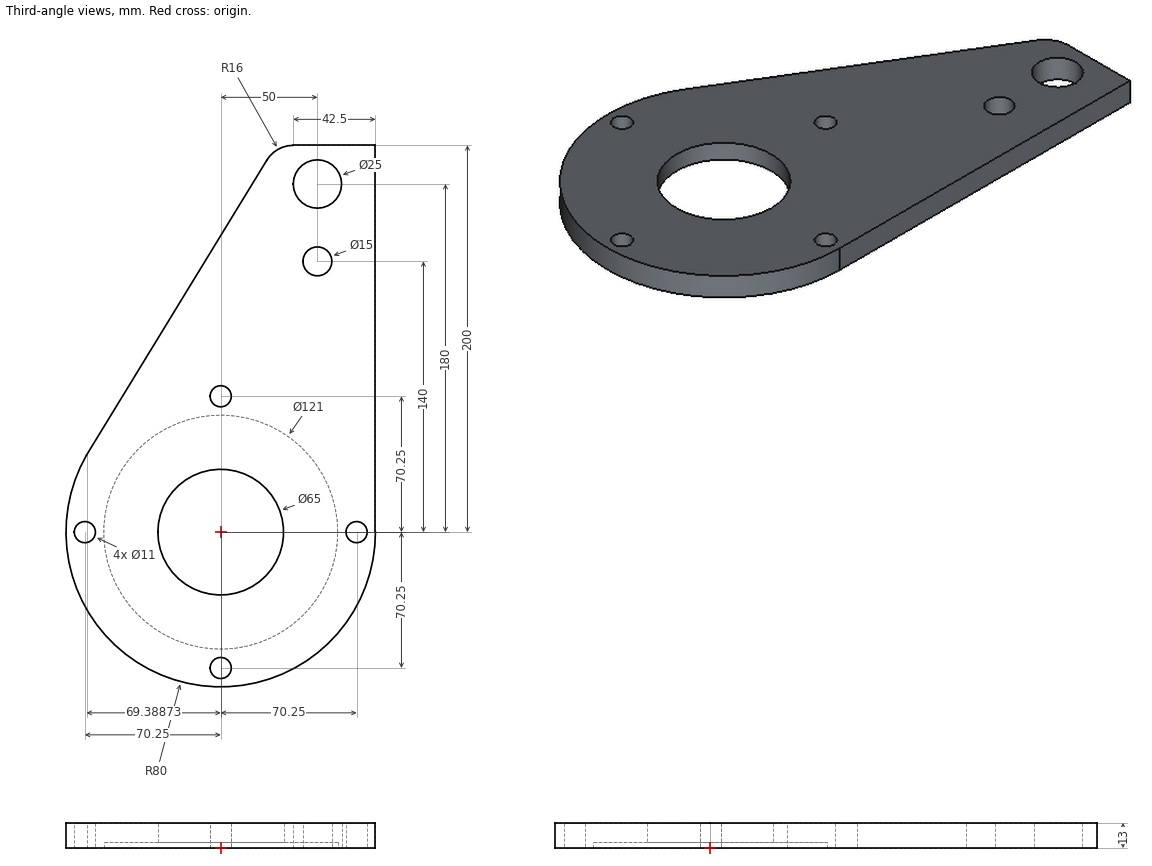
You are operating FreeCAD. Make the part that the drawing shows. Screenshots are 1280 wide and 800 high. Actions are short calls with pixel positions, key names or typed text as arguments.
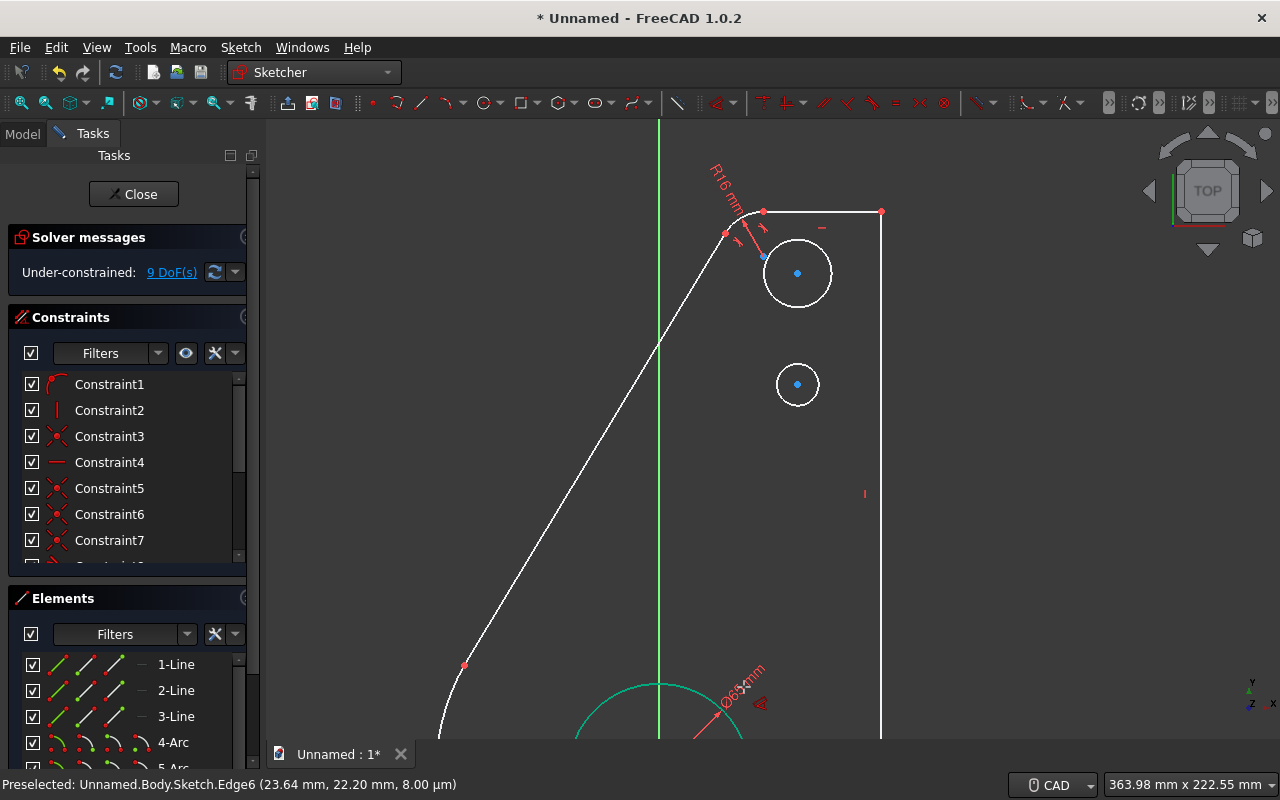
click(812, 370)
click(834, 347)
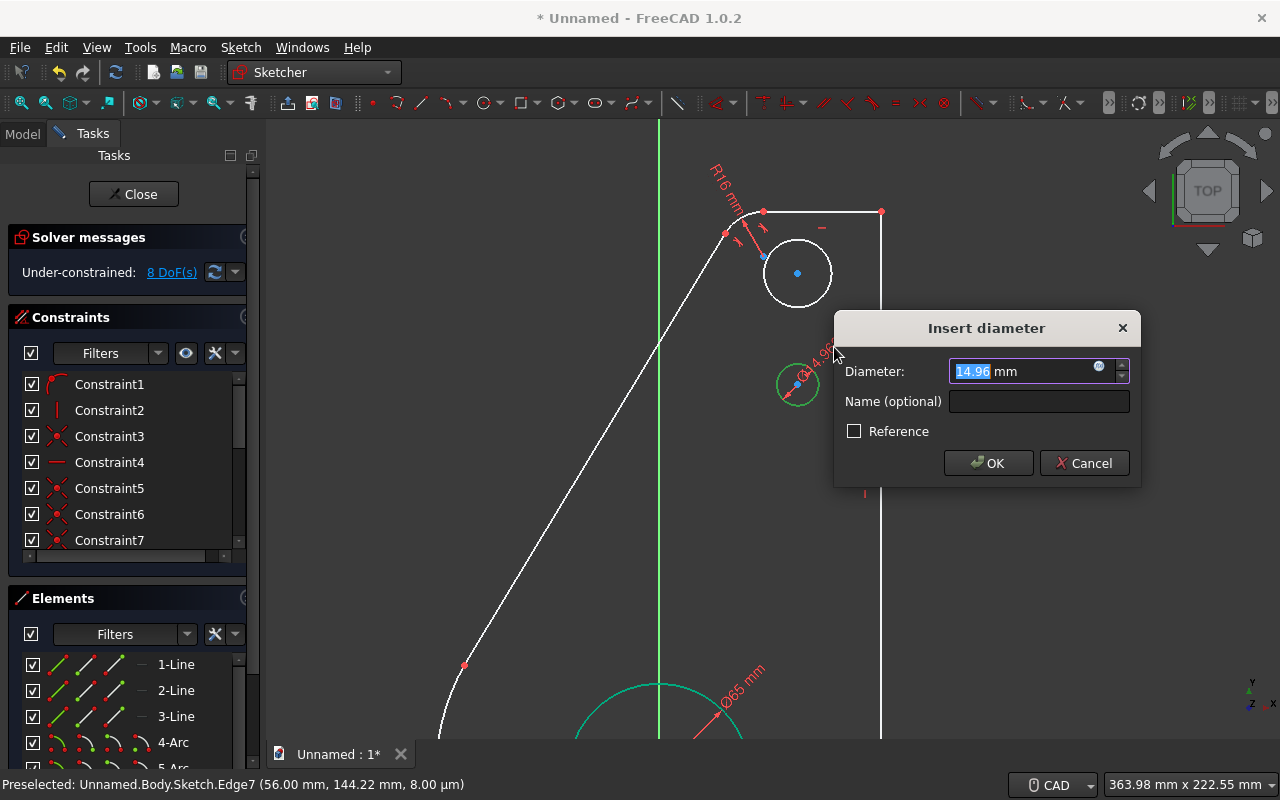
text(15)
key(Return)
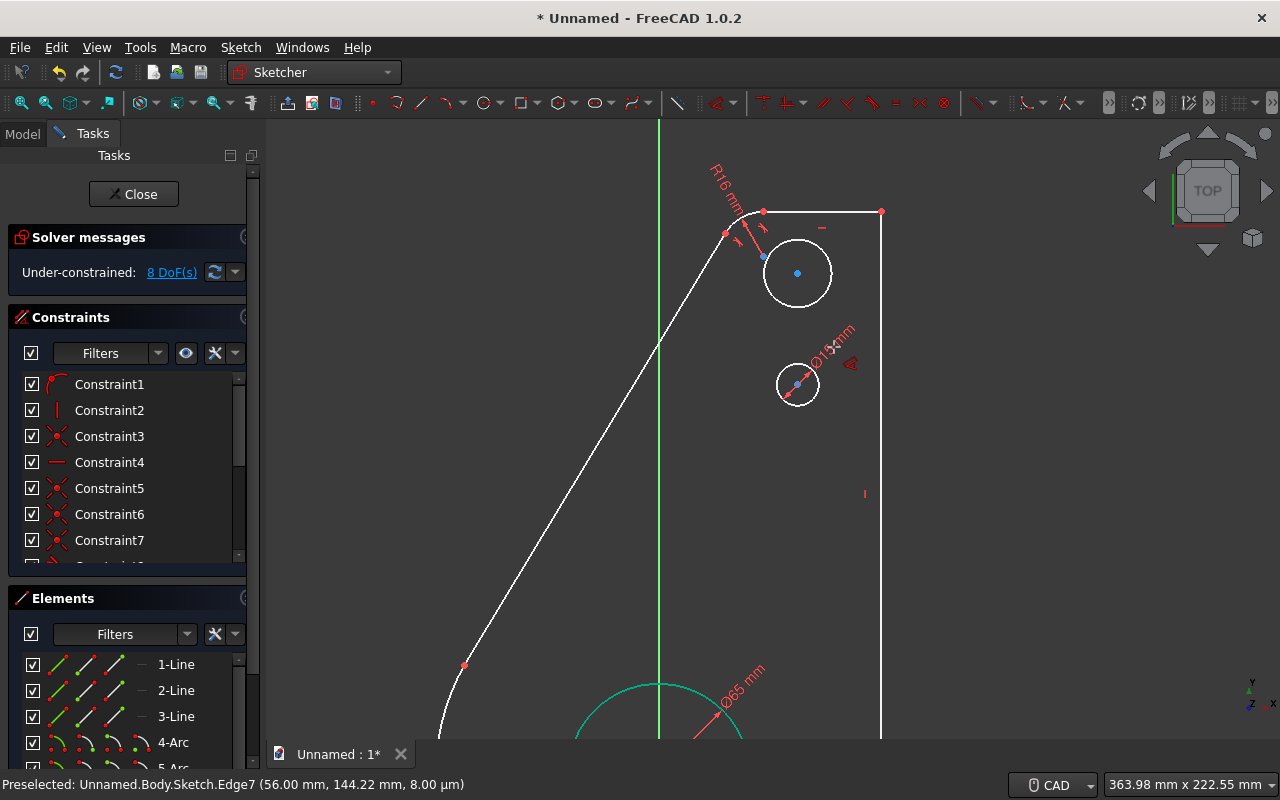
click(822, 249)
click(845, 226)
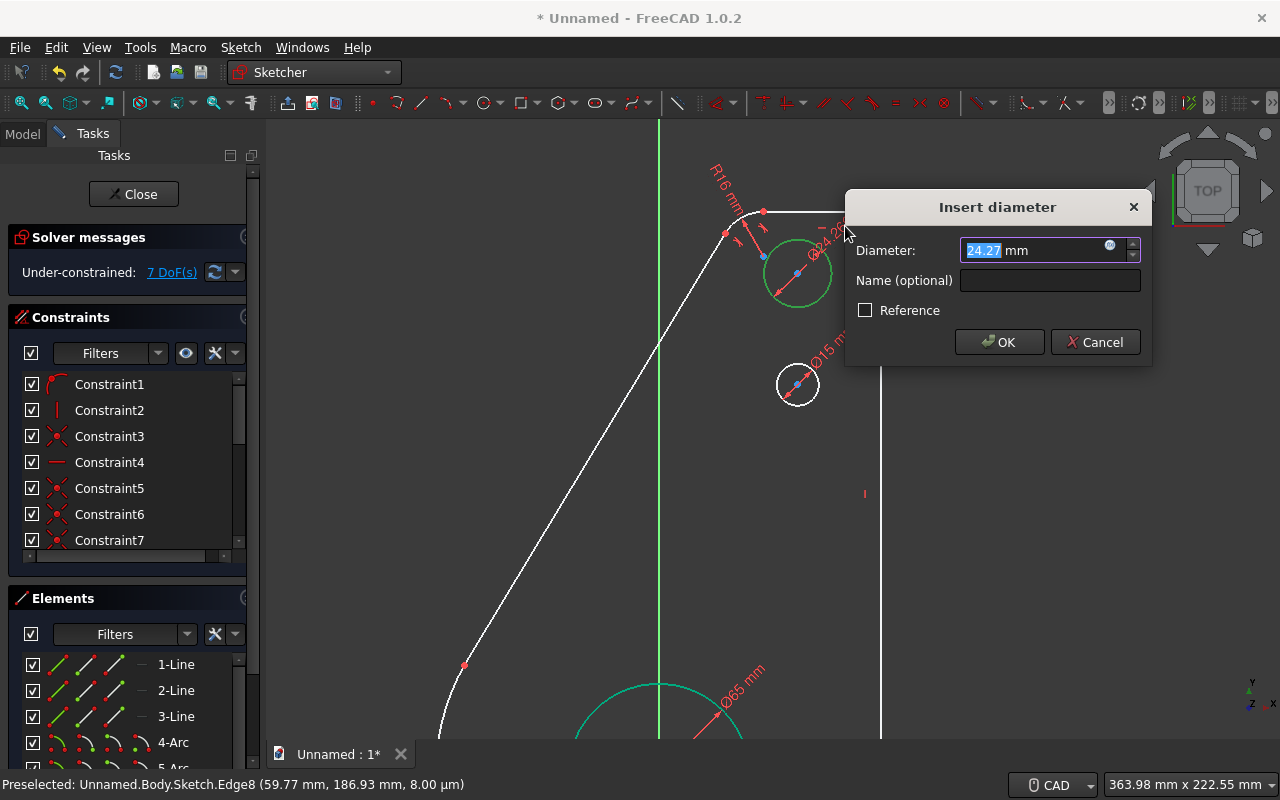
text(25)
key(Return)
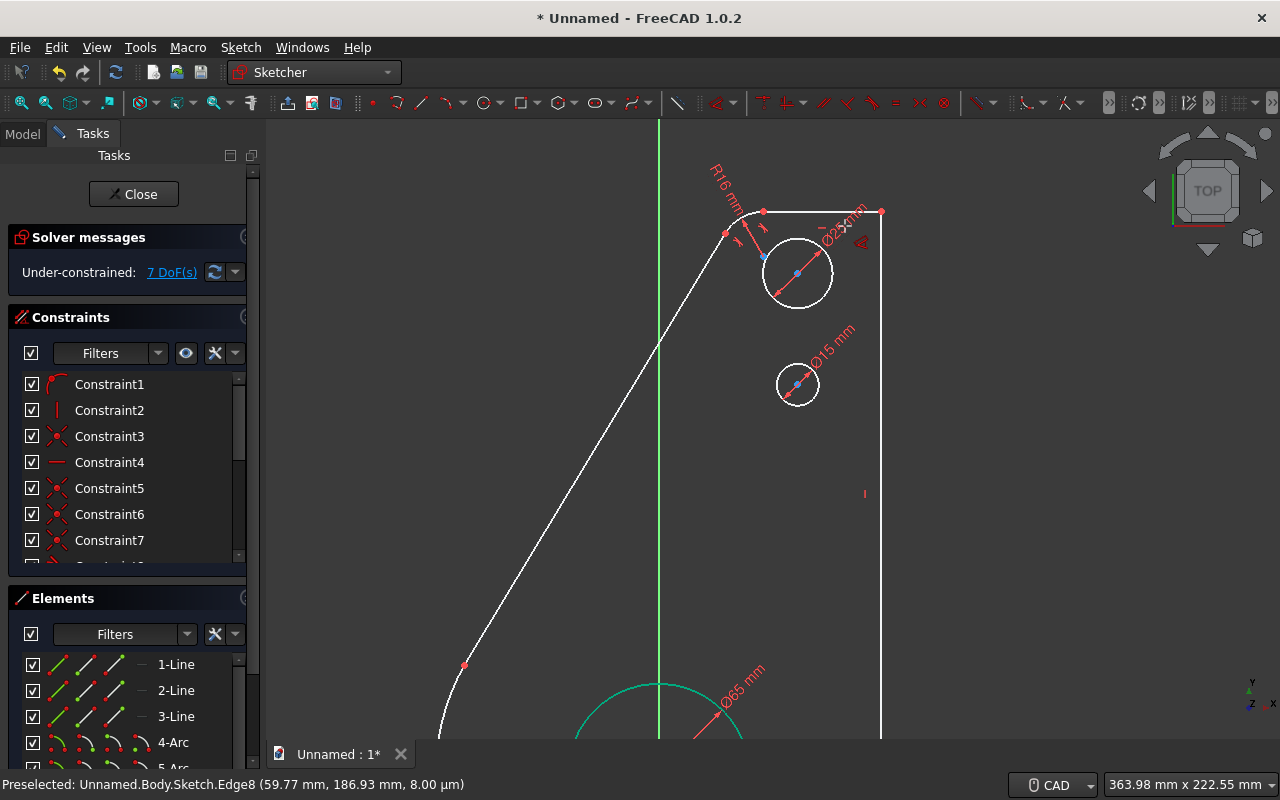
click(798, 385)
click(728, 351)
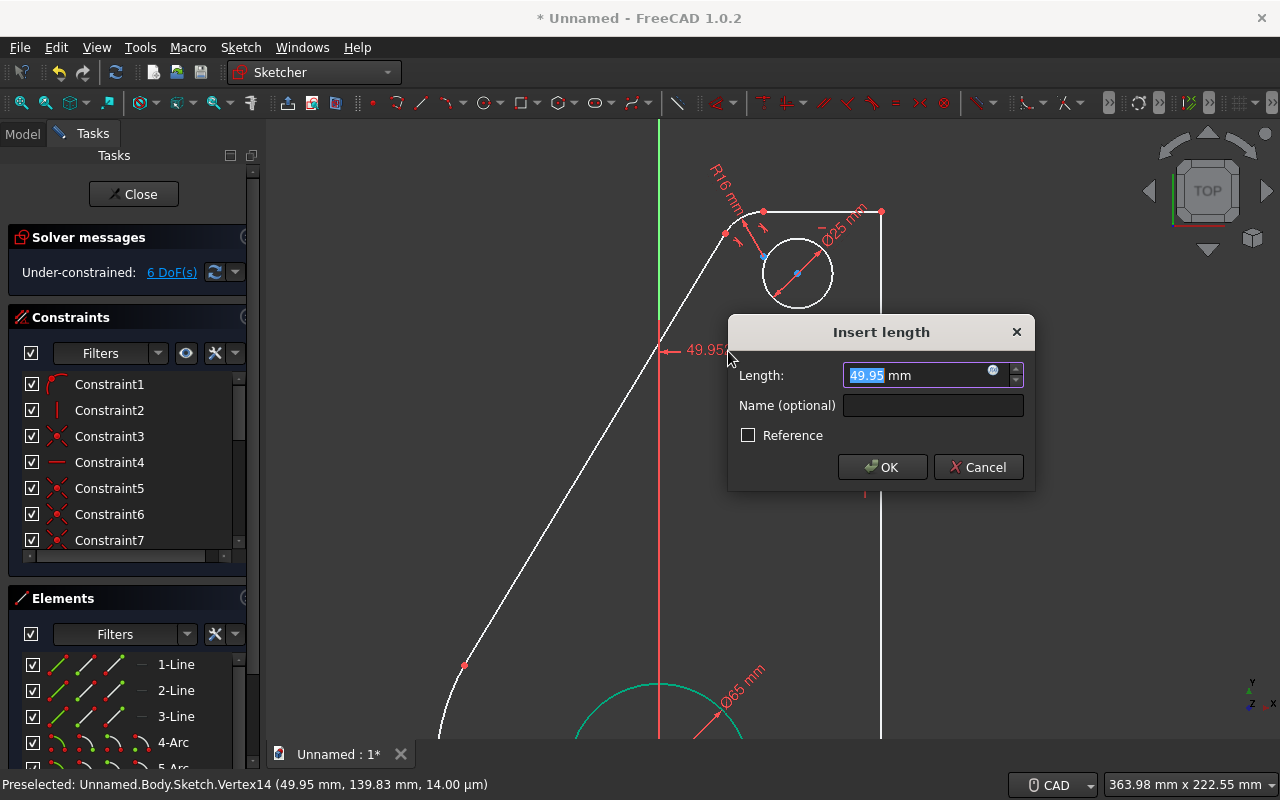
text(50)
key(Return)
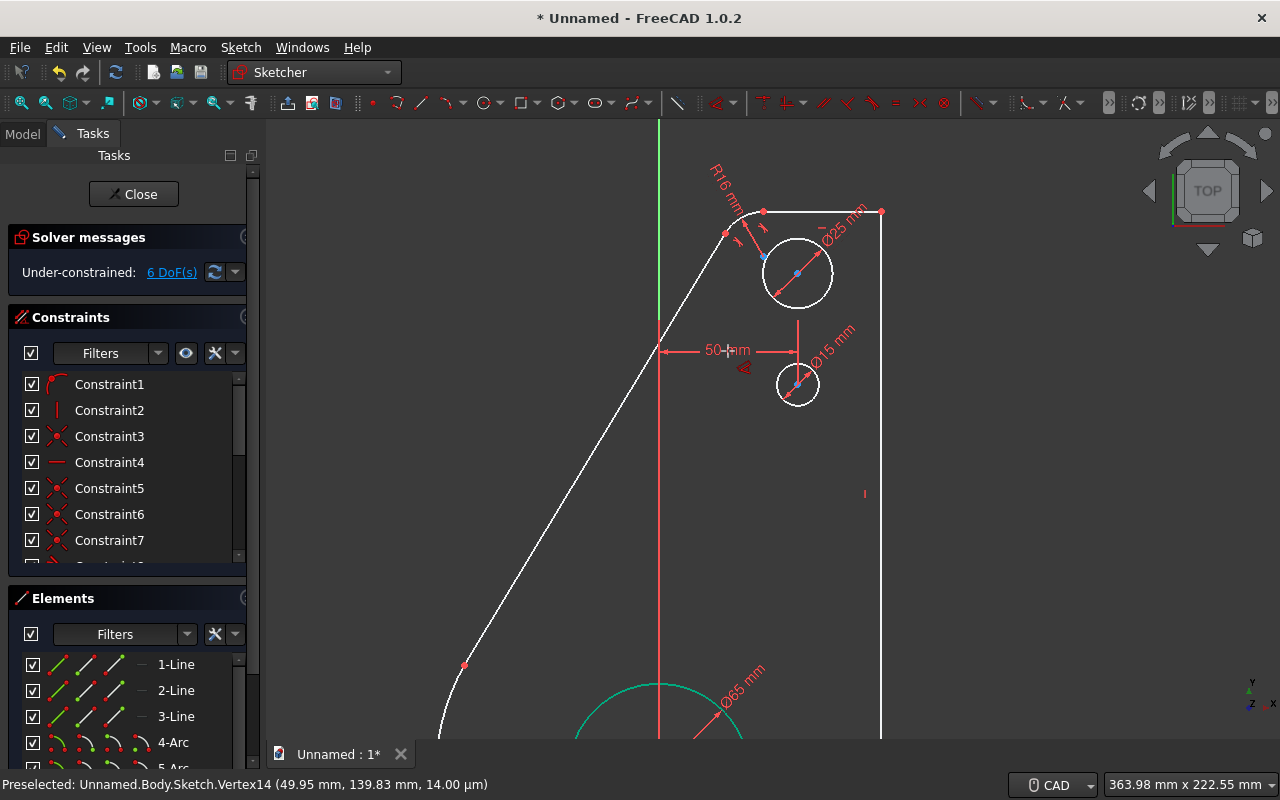
click(798, 273)
click(696, 239)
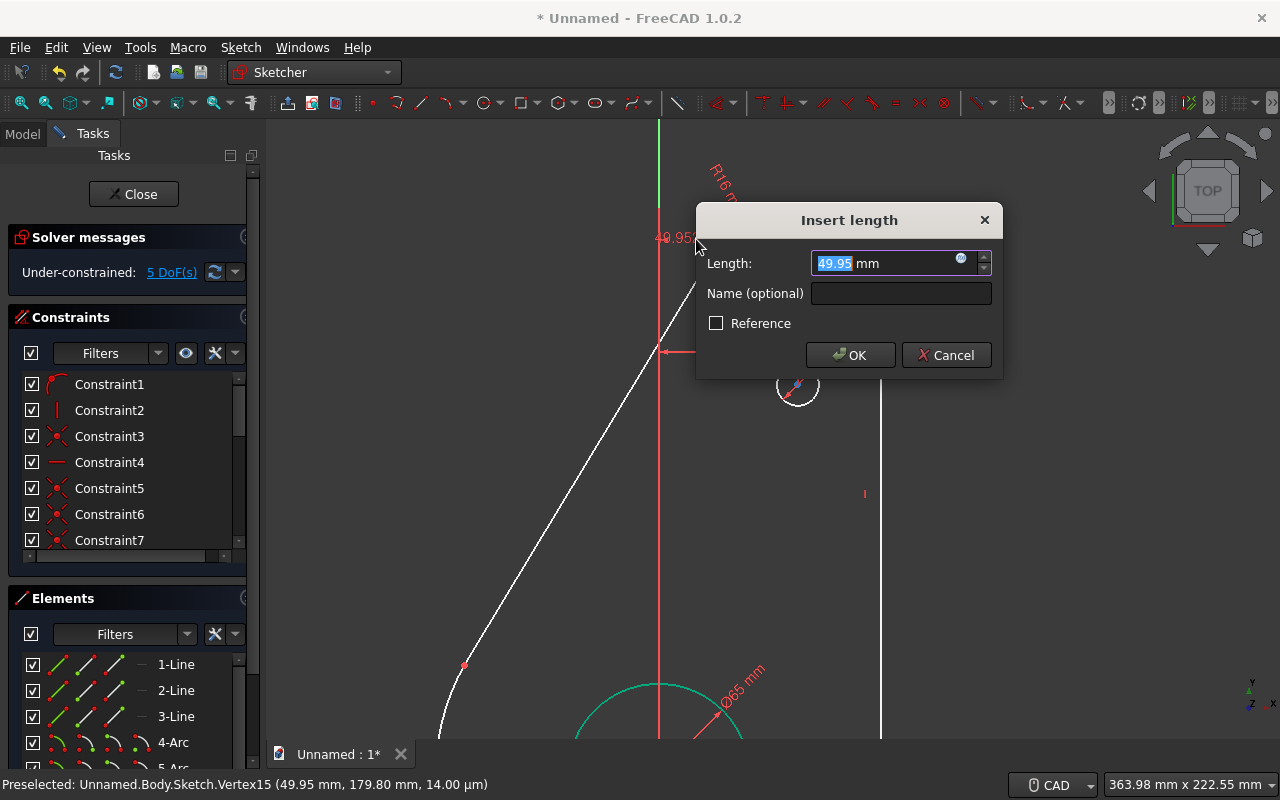
text(50)
key(Return)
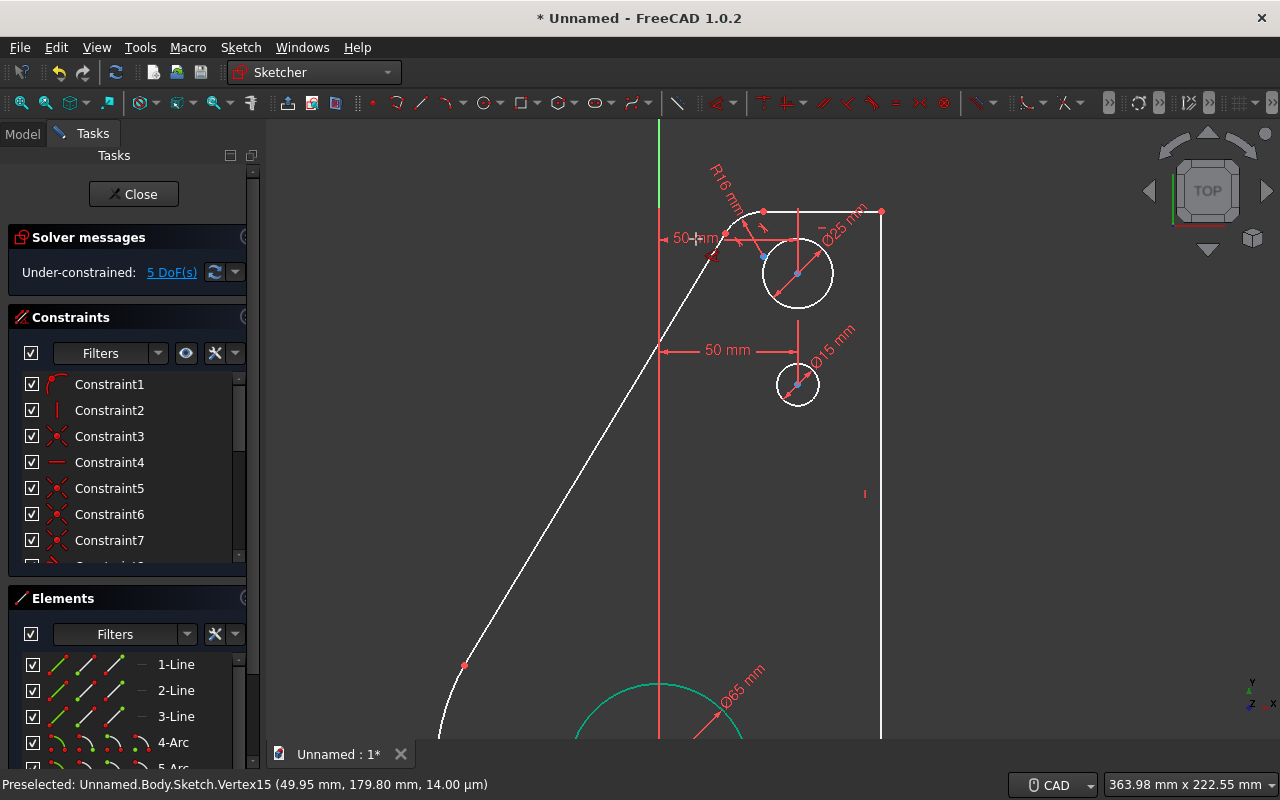
click(881, 606)
click(915, 461)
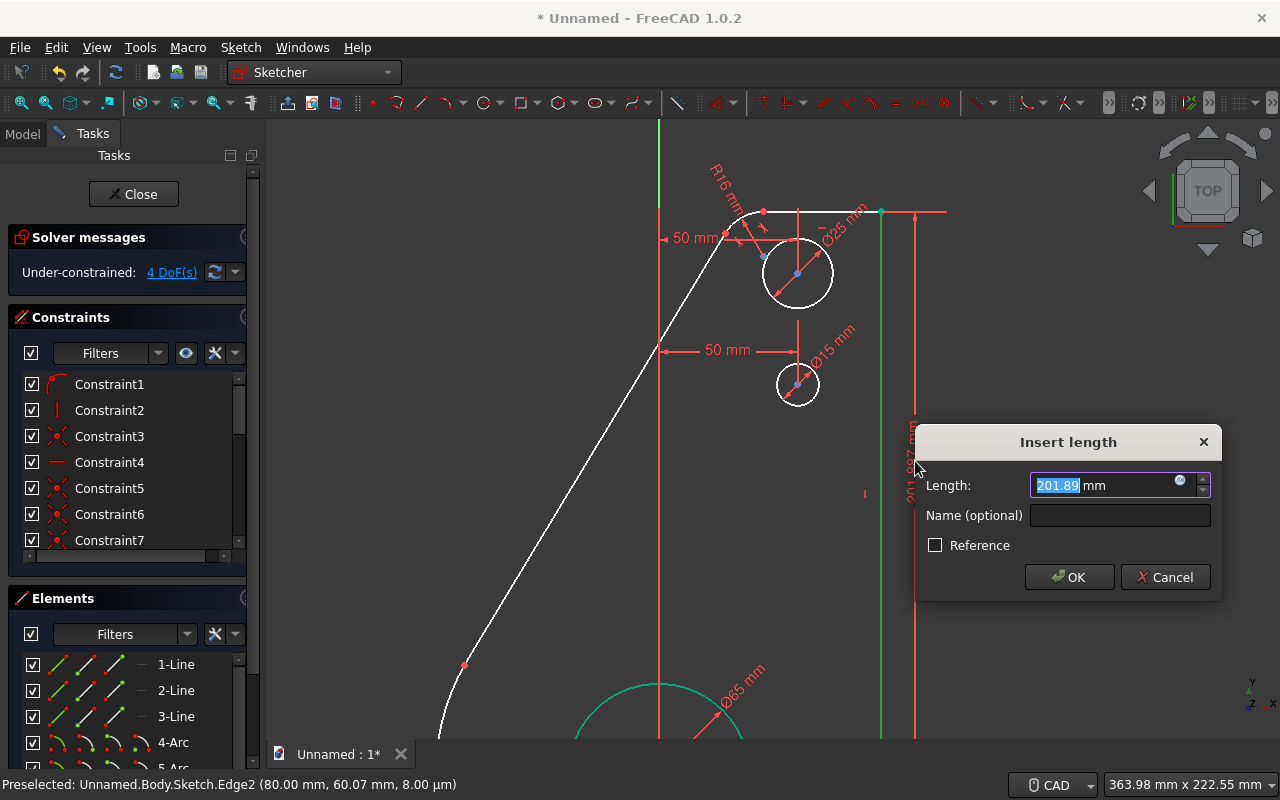
text(200)
key(Return)